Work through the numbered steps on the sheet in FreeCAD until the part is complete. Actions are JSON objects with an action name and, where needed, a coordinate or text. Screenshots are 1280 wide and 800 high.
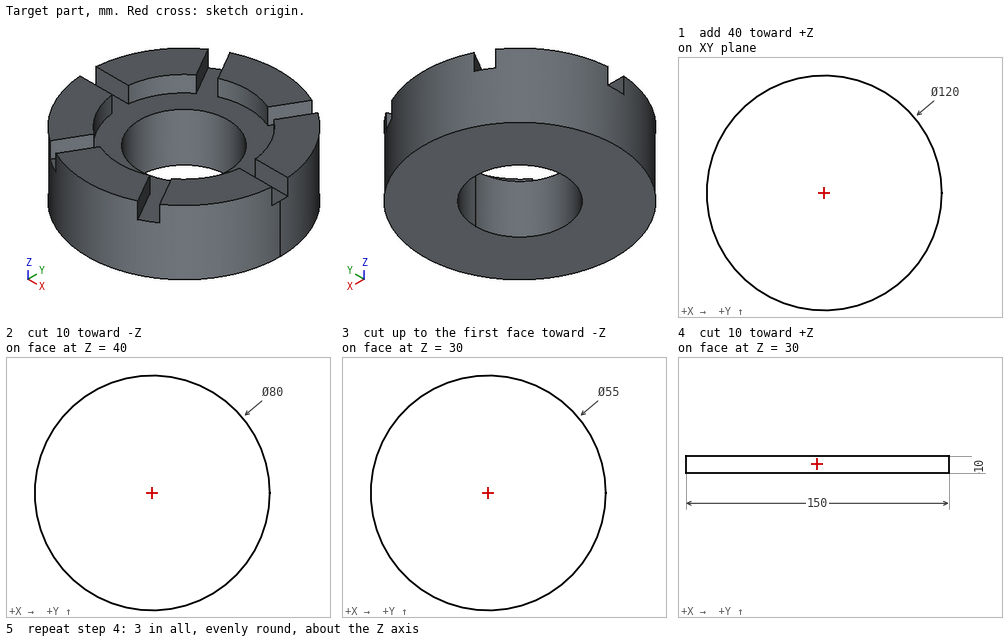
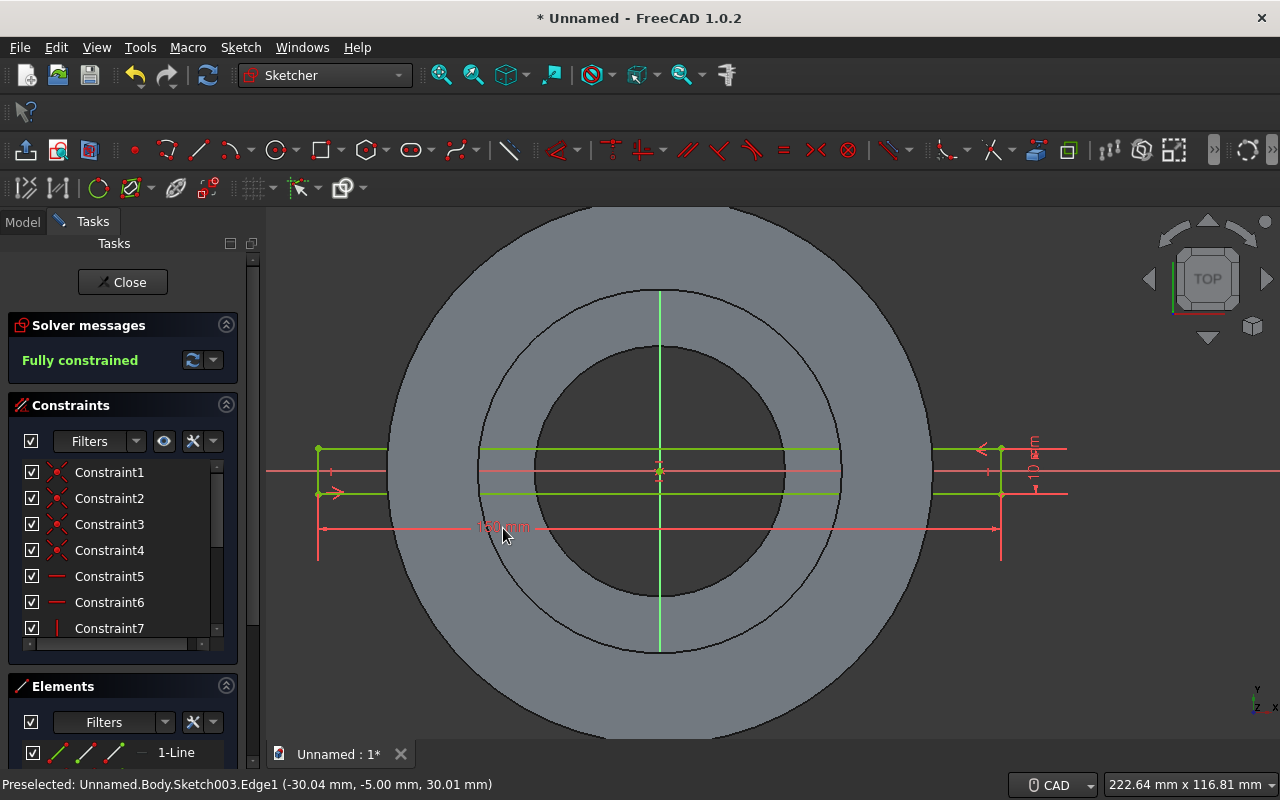
{"action": "left_click", "coordinate": [123, 282]}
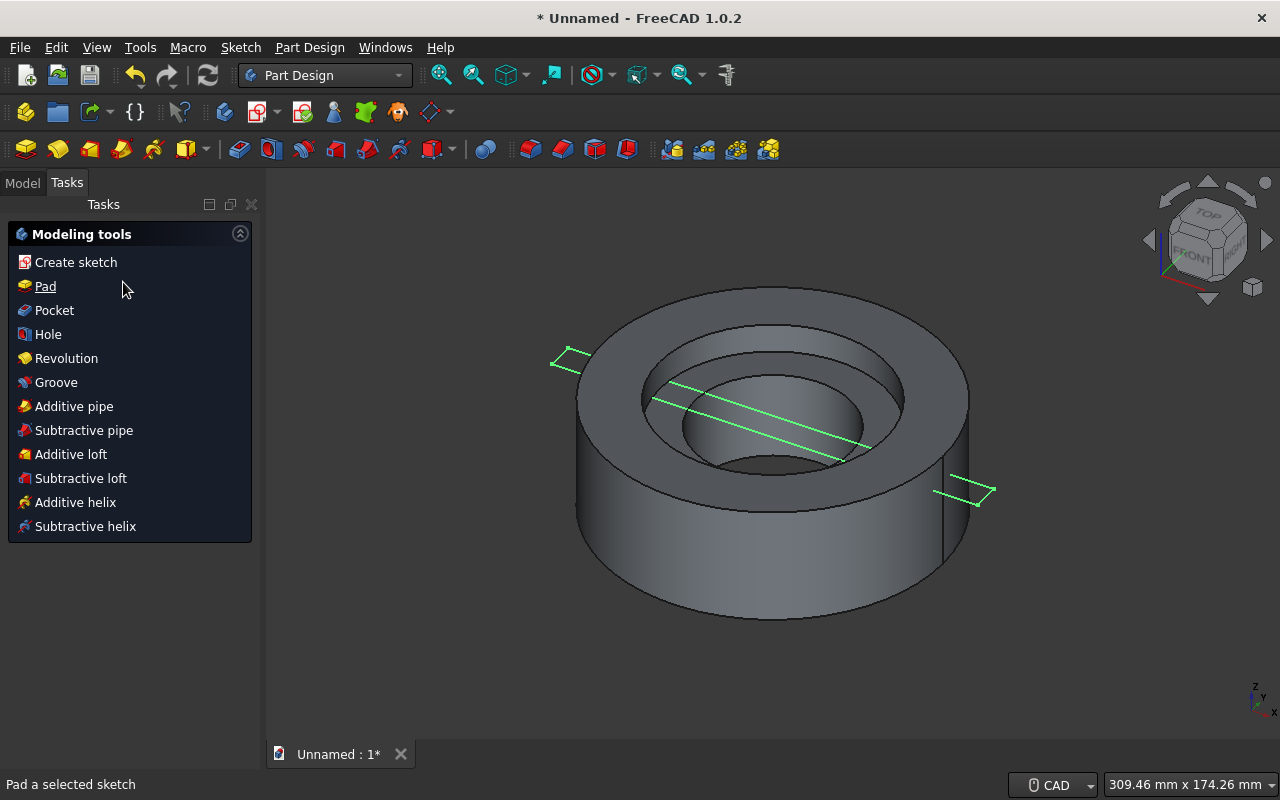
{"action": "left_click", "coordinate": [240, 150]}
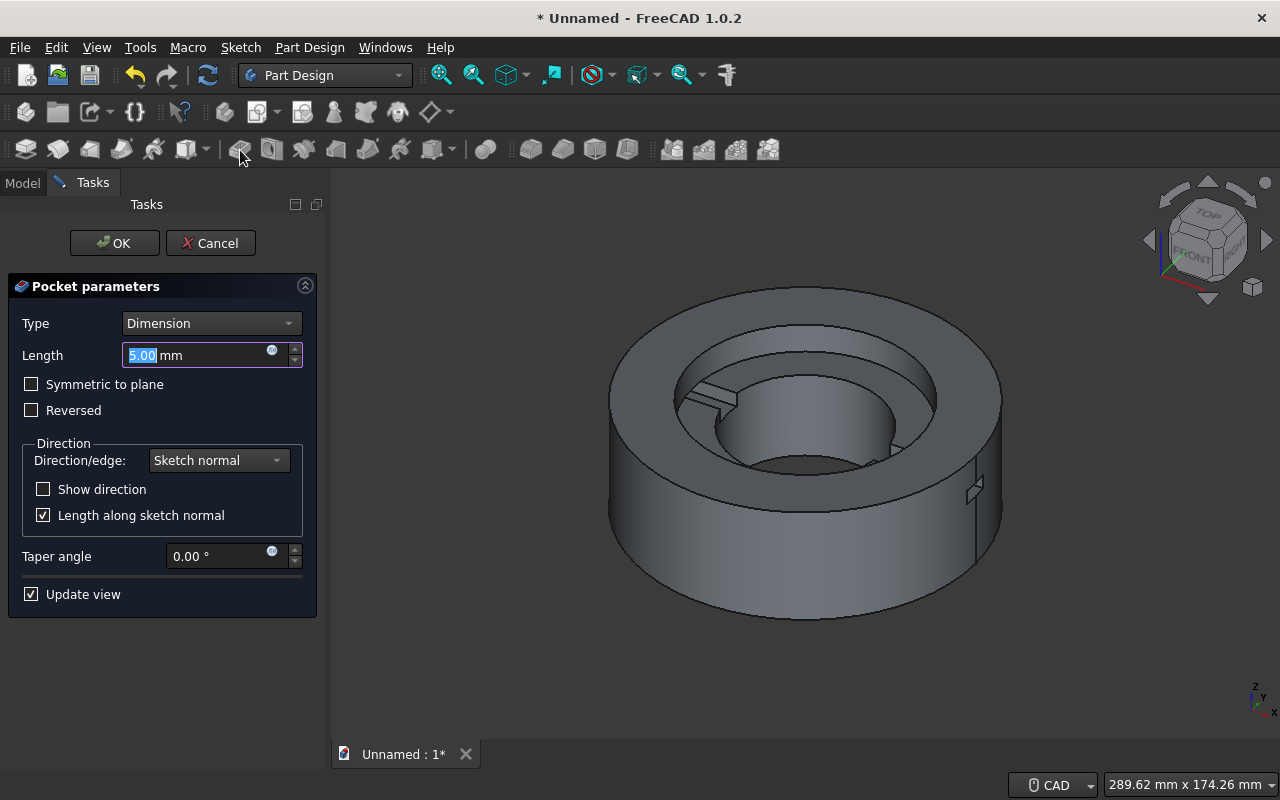
{"action": "type", "text": "10"}
{"action": "key", "text": "Tab"}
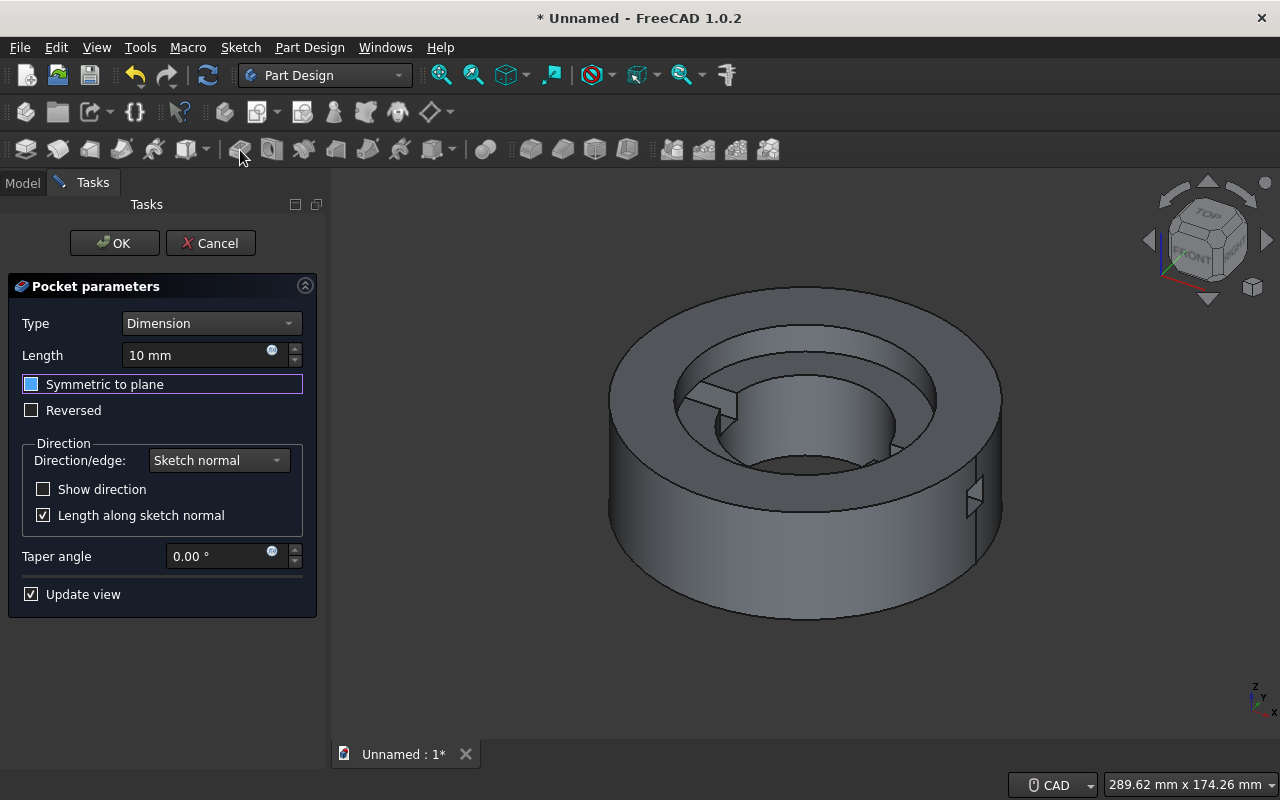
{"action": "left_click", "coordinate": [30, 410]}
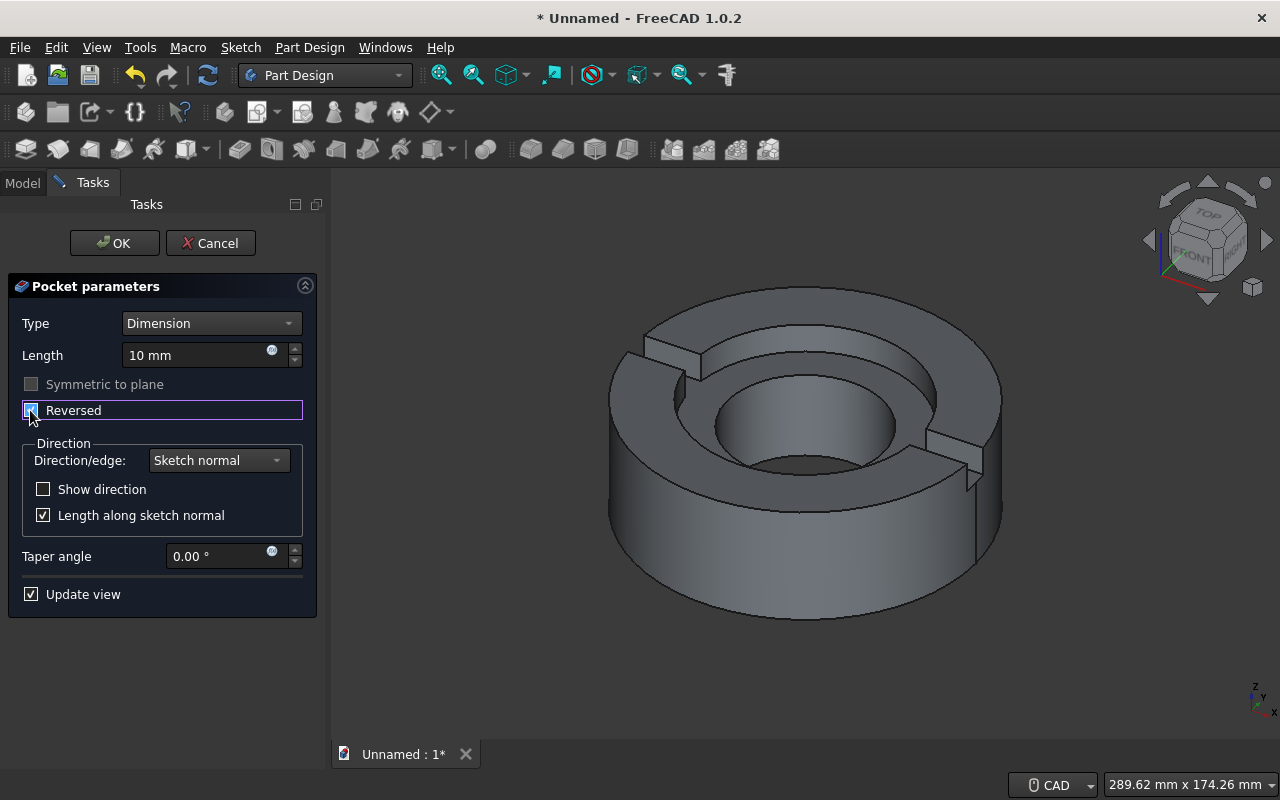
{"action": "left_click", "coordinate": [115, 243]}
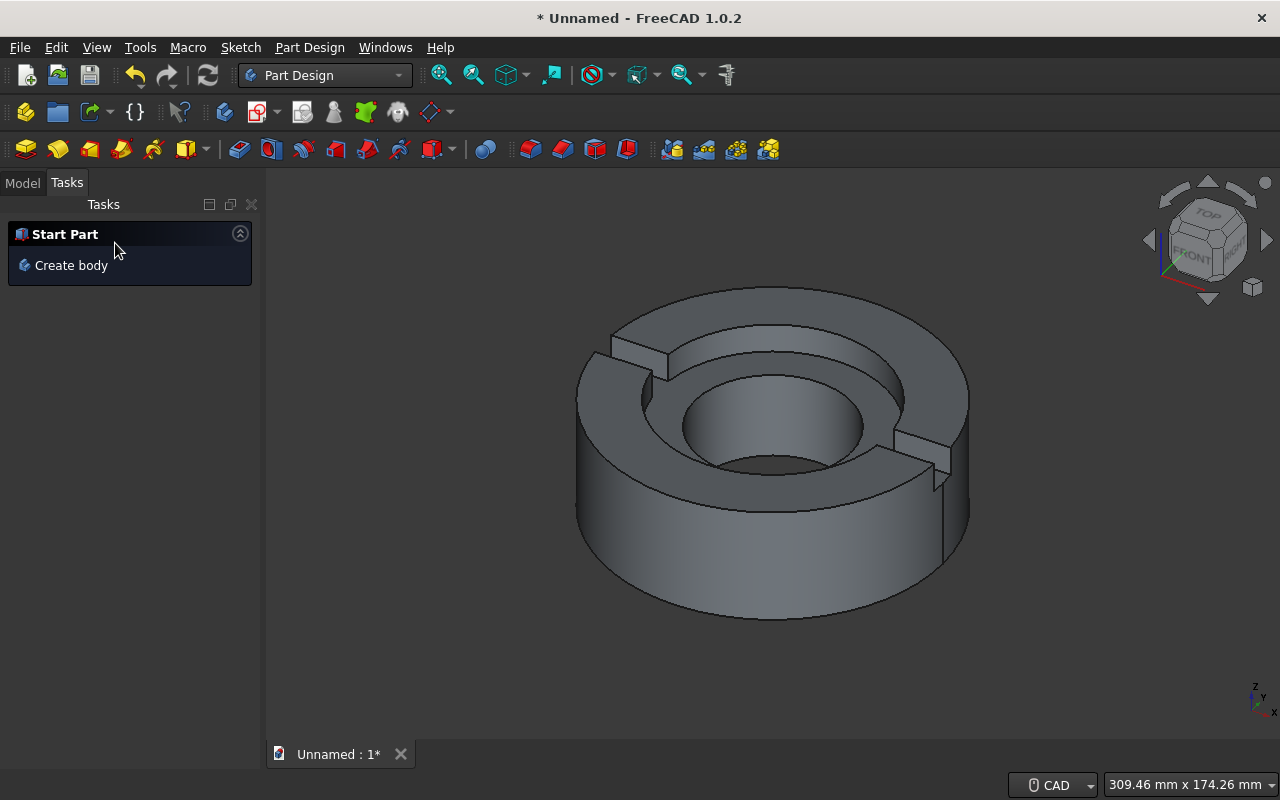
{"action": "left_click", "coordinate": [23, 182]}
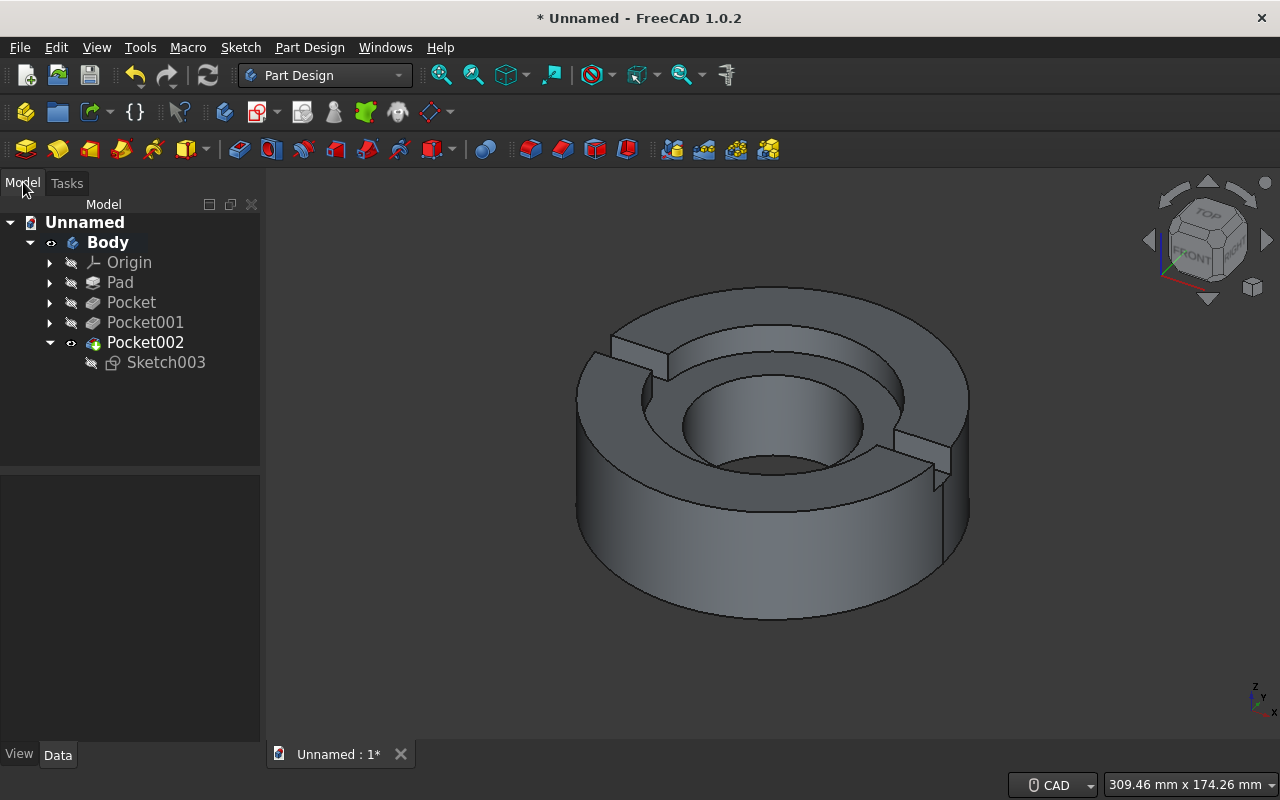
{"action": "left_click", "coordinate": [116, 343]}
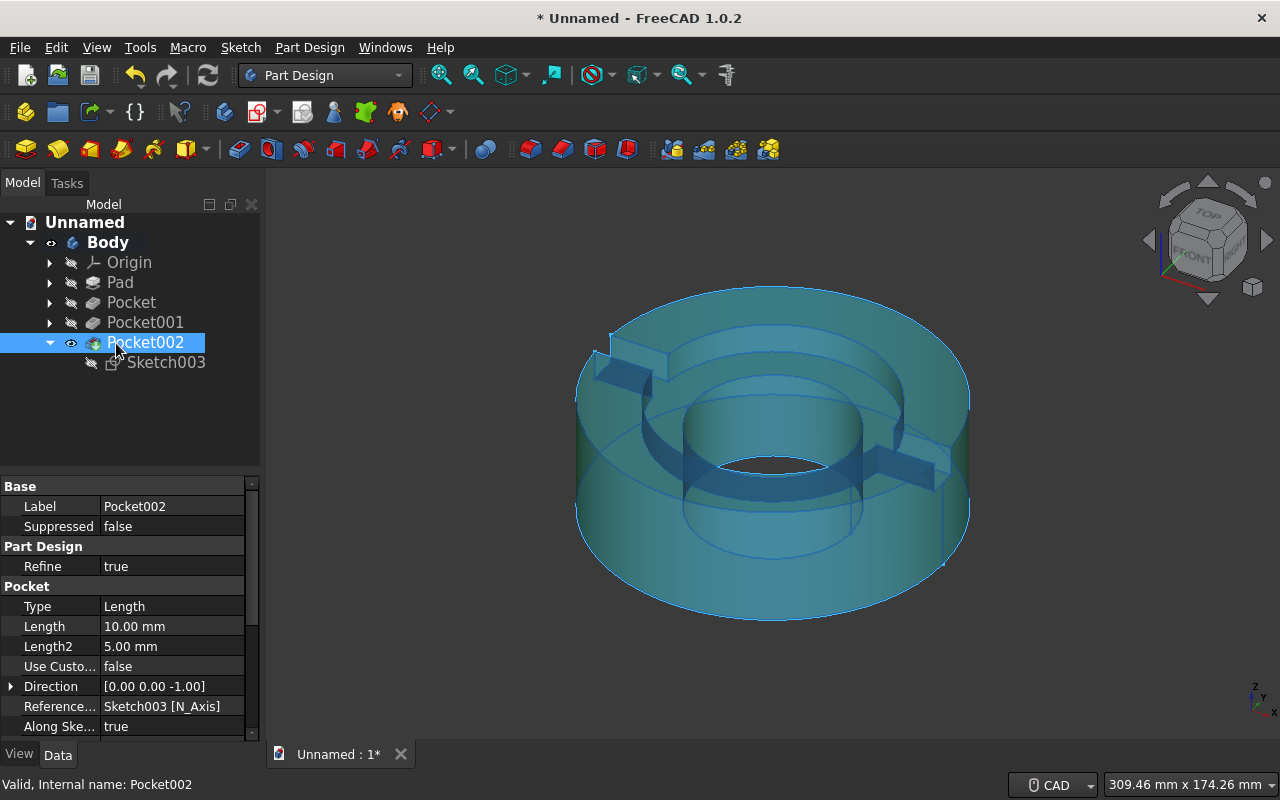
{"action": "left_click", "coordinate": [736, 150]}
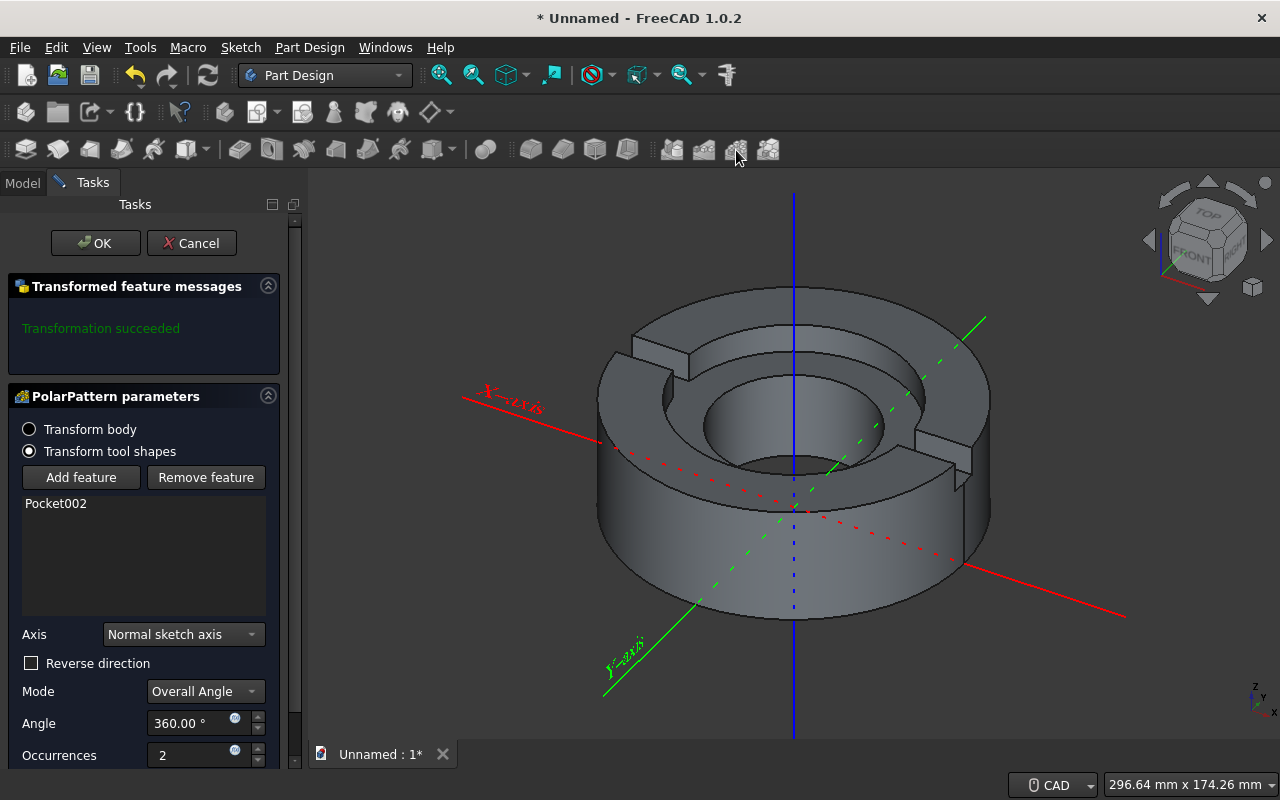
{"action": "left_click", "coordinate": [184, 634]}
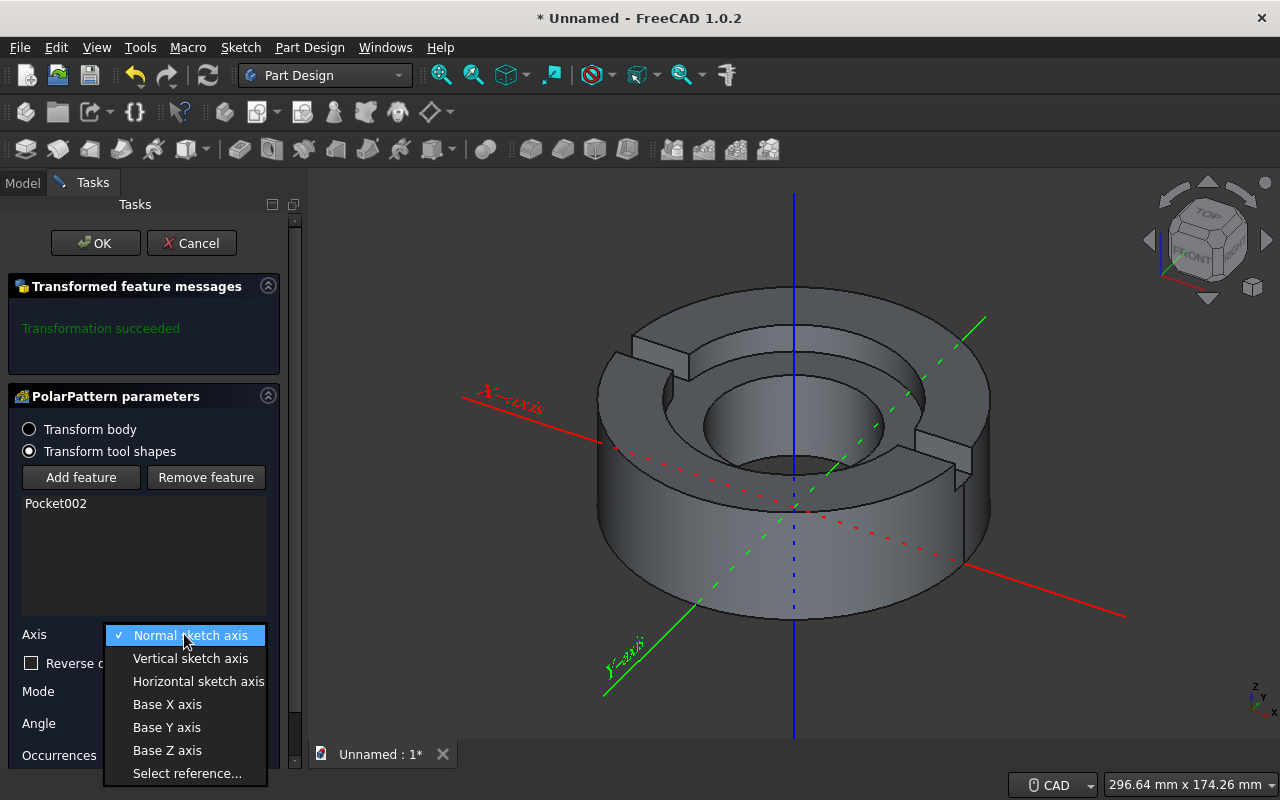
{"action": "left_click", "coordinate": [184, 750]}